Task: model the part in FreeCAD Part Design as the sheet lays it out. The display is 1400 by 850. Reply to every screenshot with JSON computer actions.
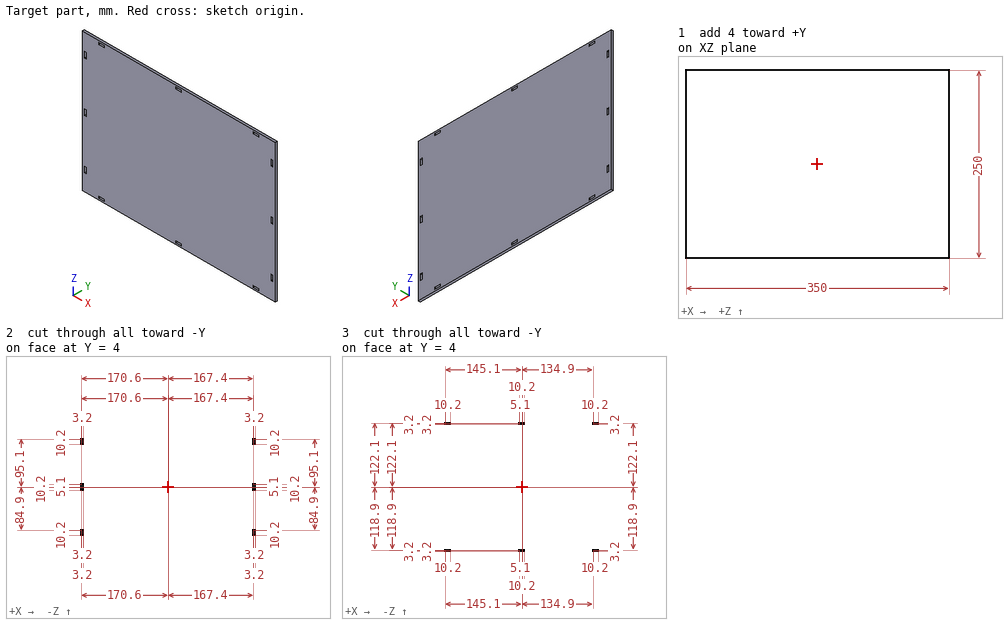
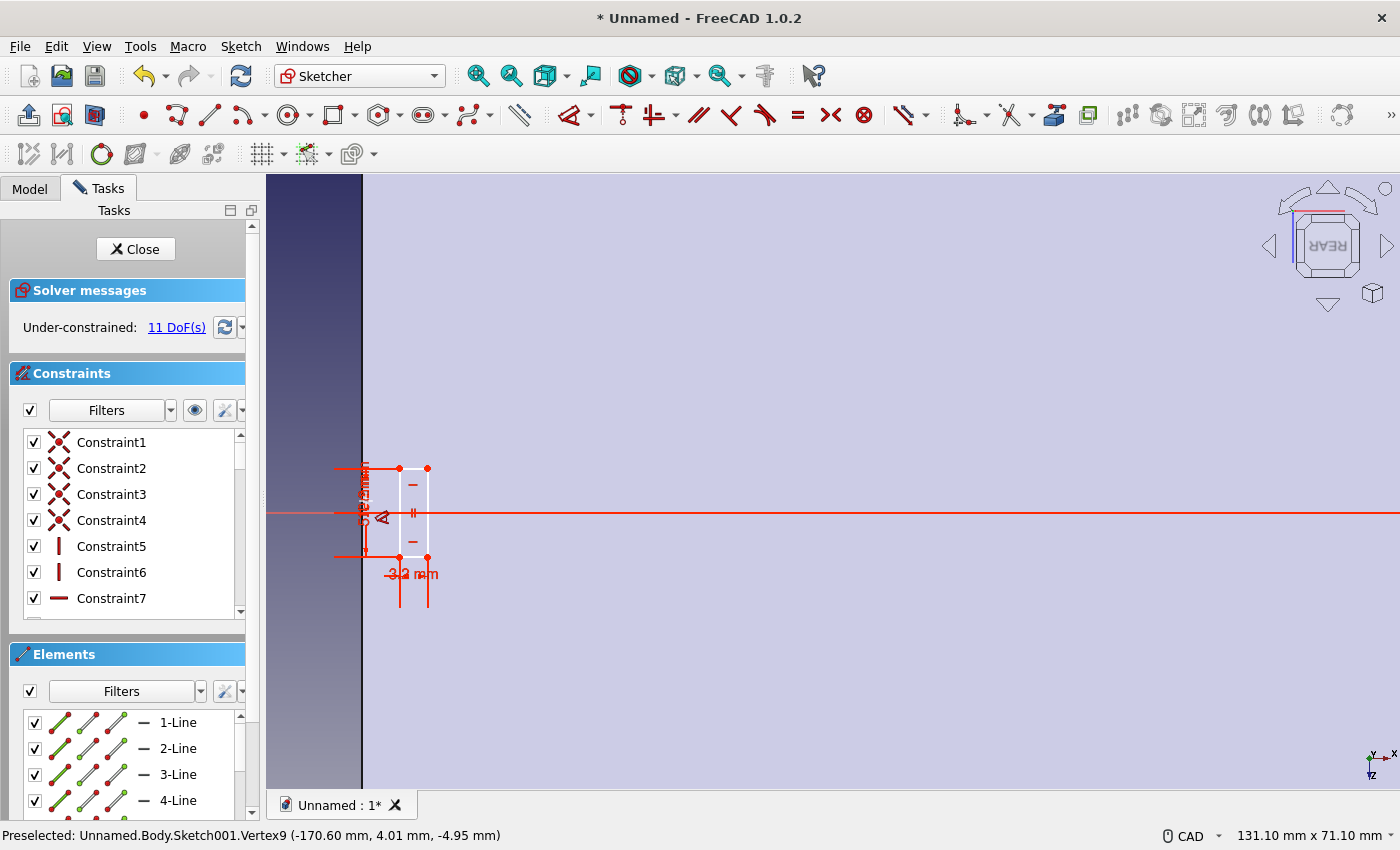
{"action": "scroll", "coordinate": [401, 471], "scroll_direction": "down", "scroll_amount": 7}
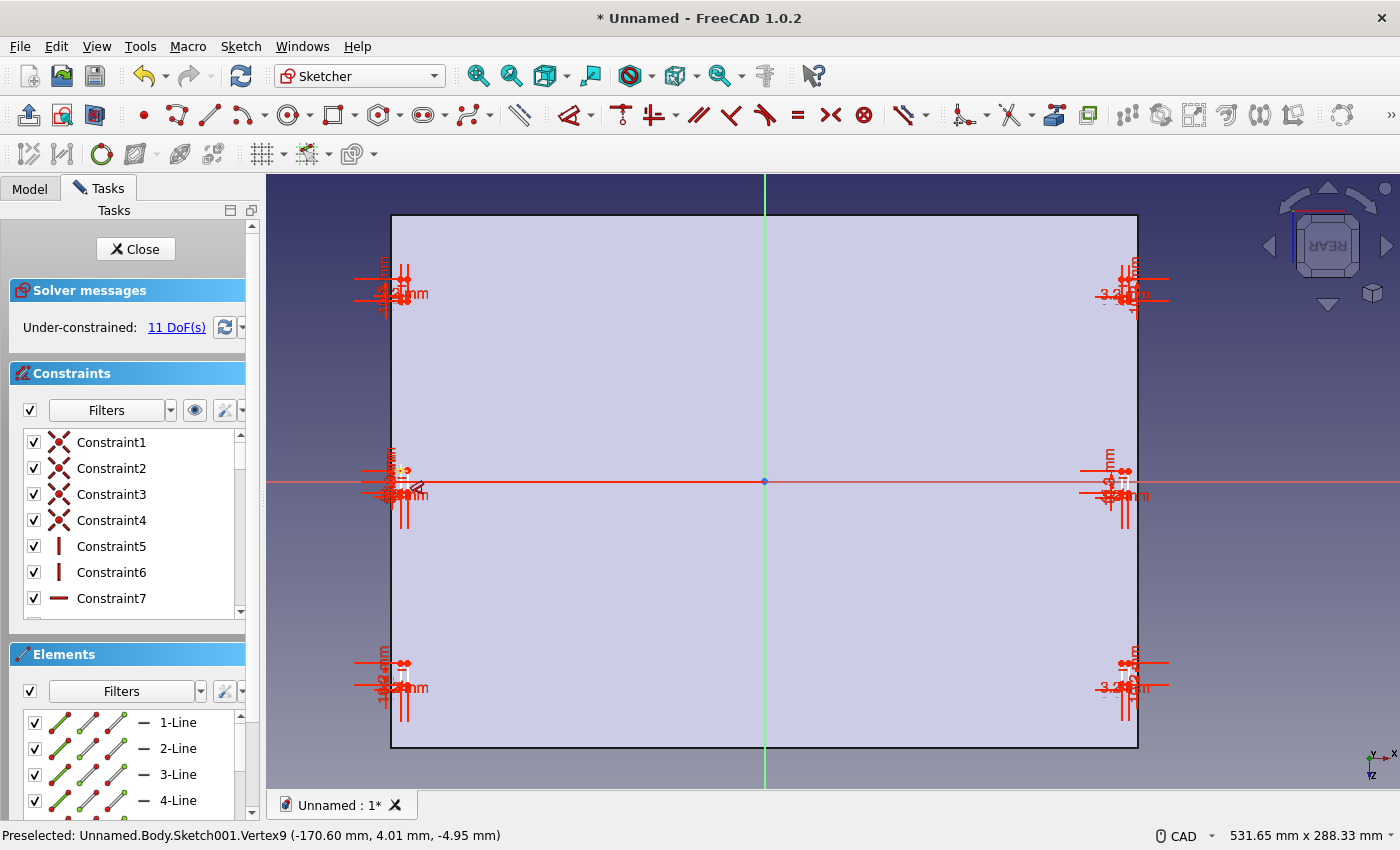
{"action": "scroll", "coordinate": [1122, 471], "scroll_direction": "up", "scroll_amount": 7}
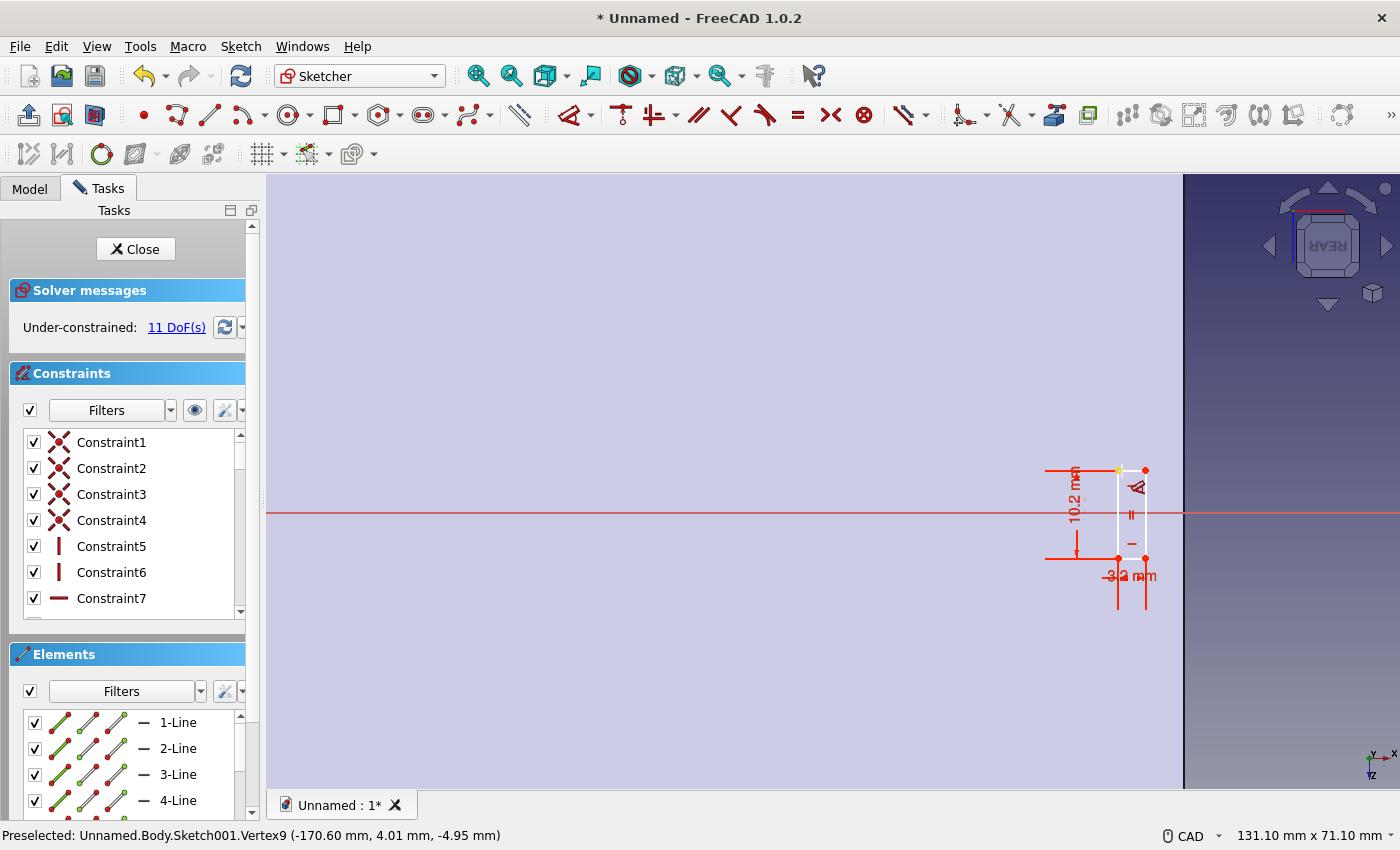
{"action": "left_click", "coordinate": [1118, 471]}
{"action": "left_click", "coordinate": [1176, 492]}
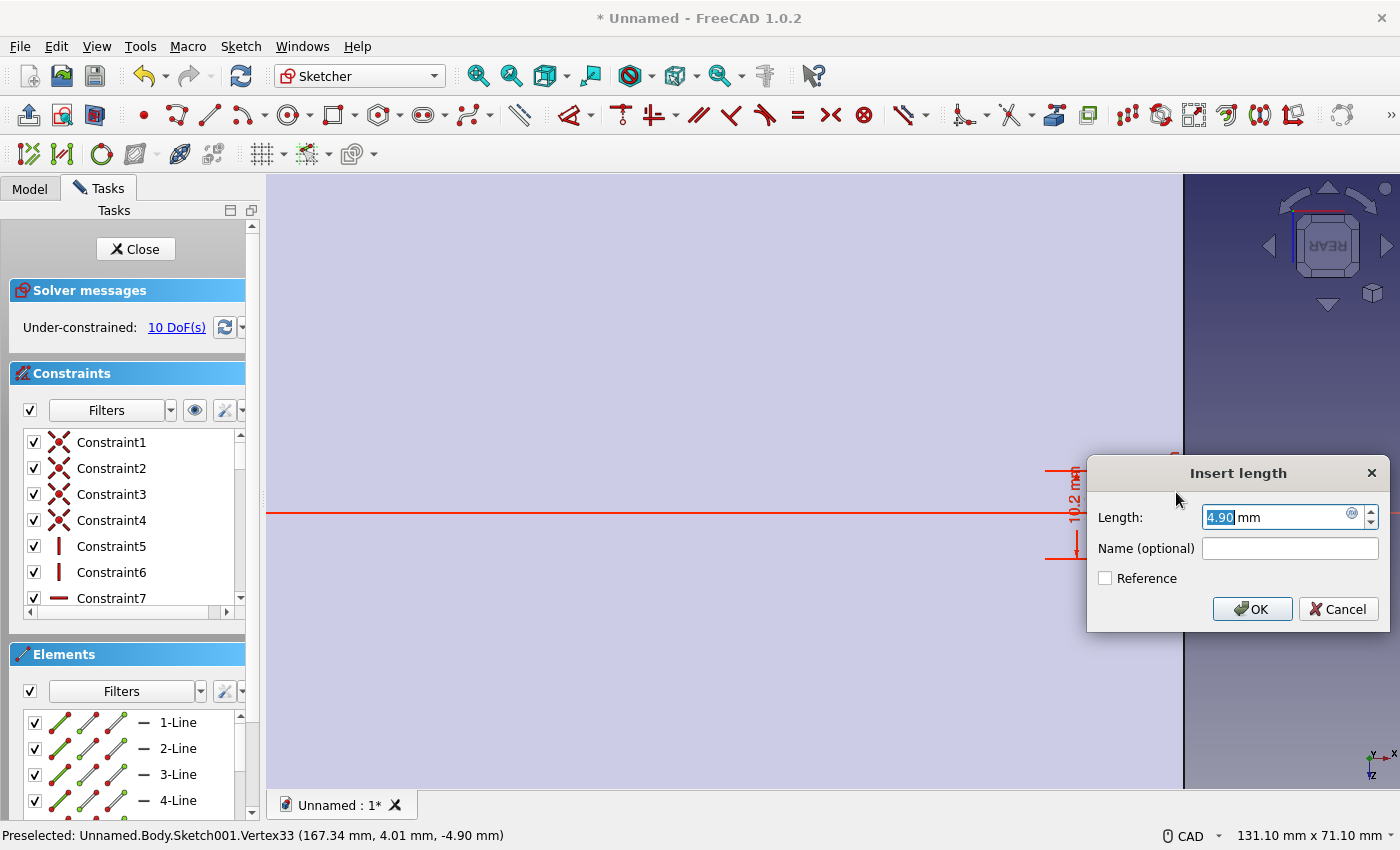
{"action": "type", "text": "5.1"}
{"action": "key", "text": "Return"}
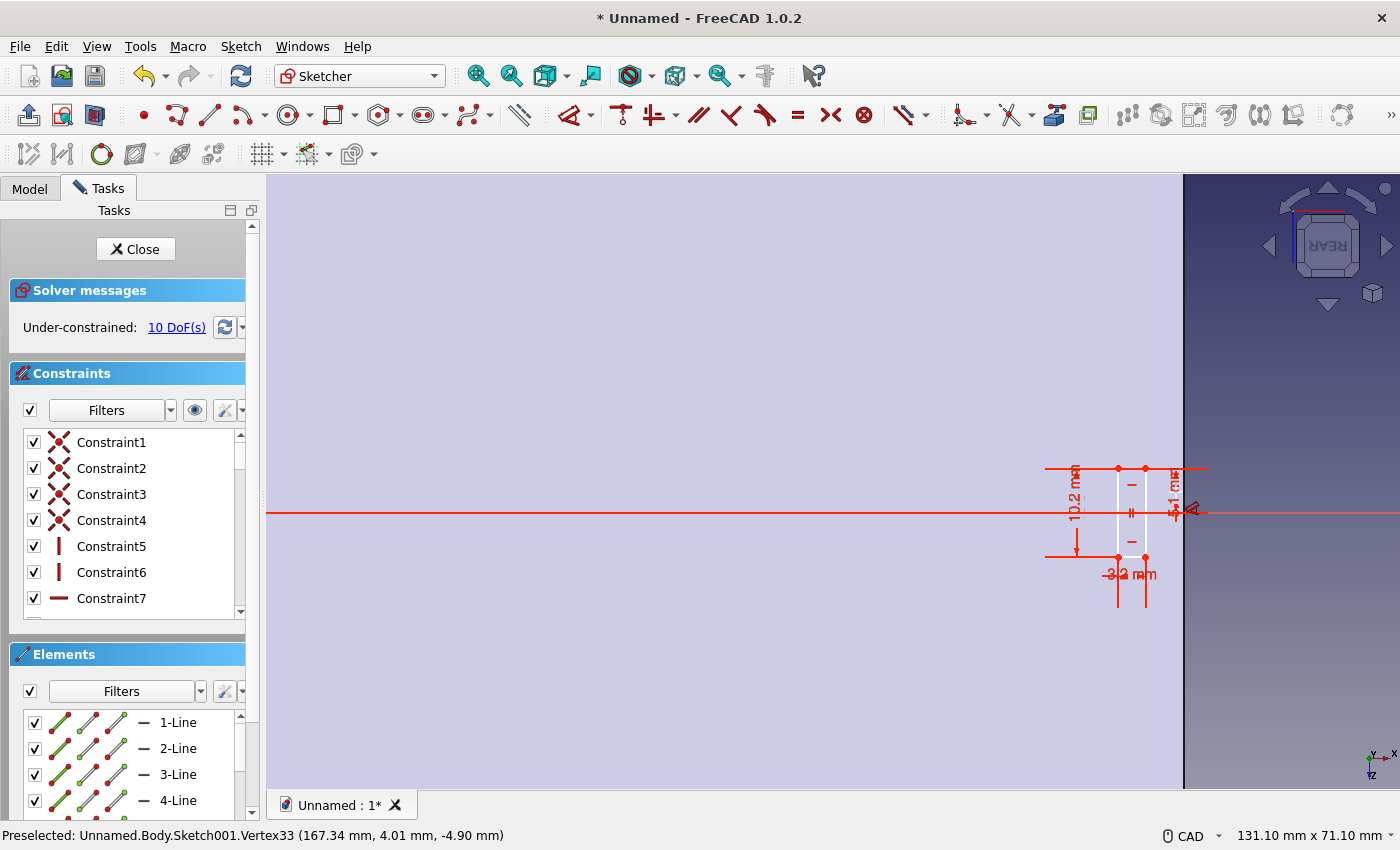
{"action": "scroll", "coordinate": [1122, 471], "scroll_direction": "down", "scroll_amount": 7}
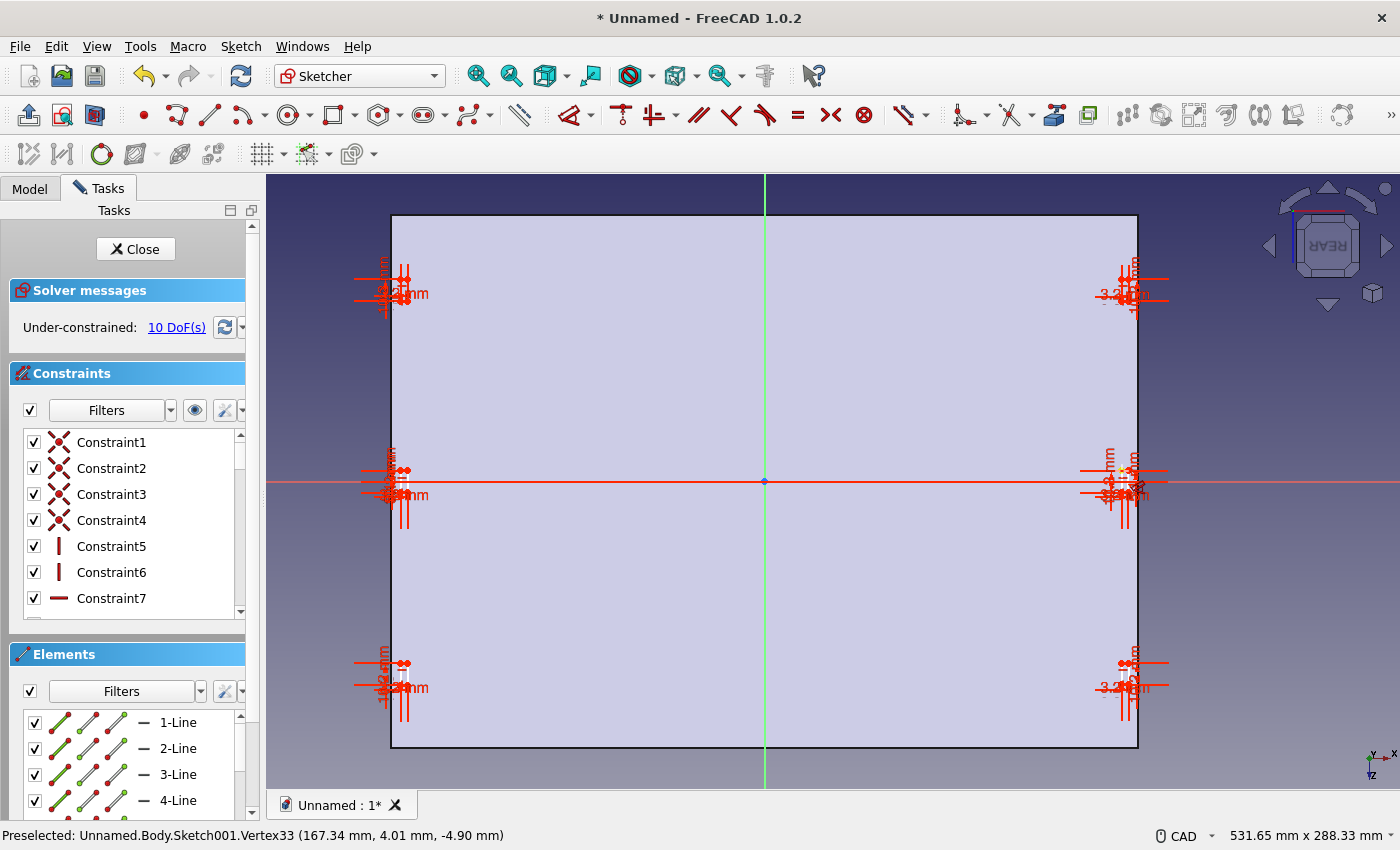
{"action": "scroll", "coordinate": [401, 279], "scroll_direction": "up", "scroll_amount": 3}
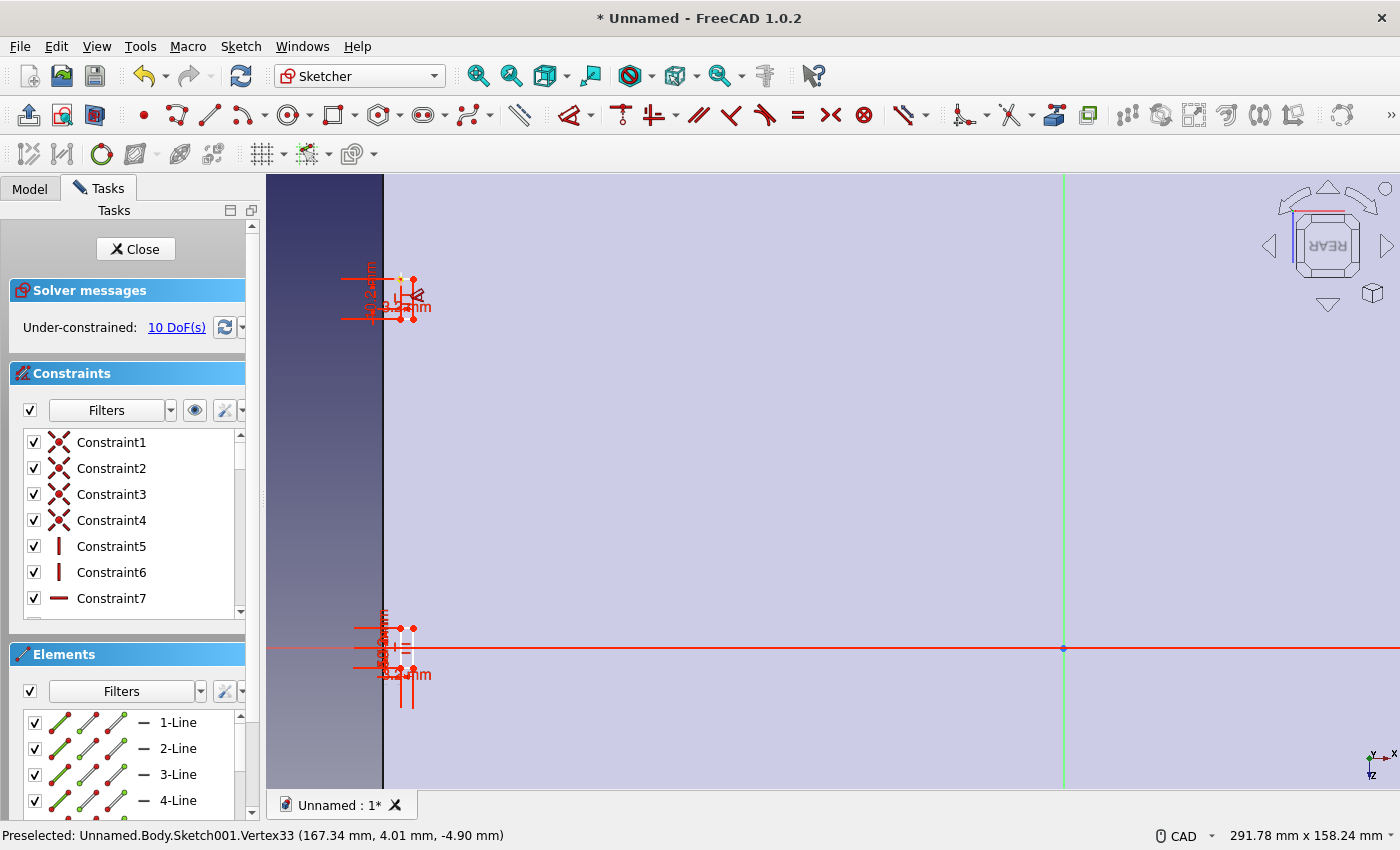
{"action": "left_click", "coordinate": [401, 279]}
{"action": "left_click", "coordinate": [367, 464]}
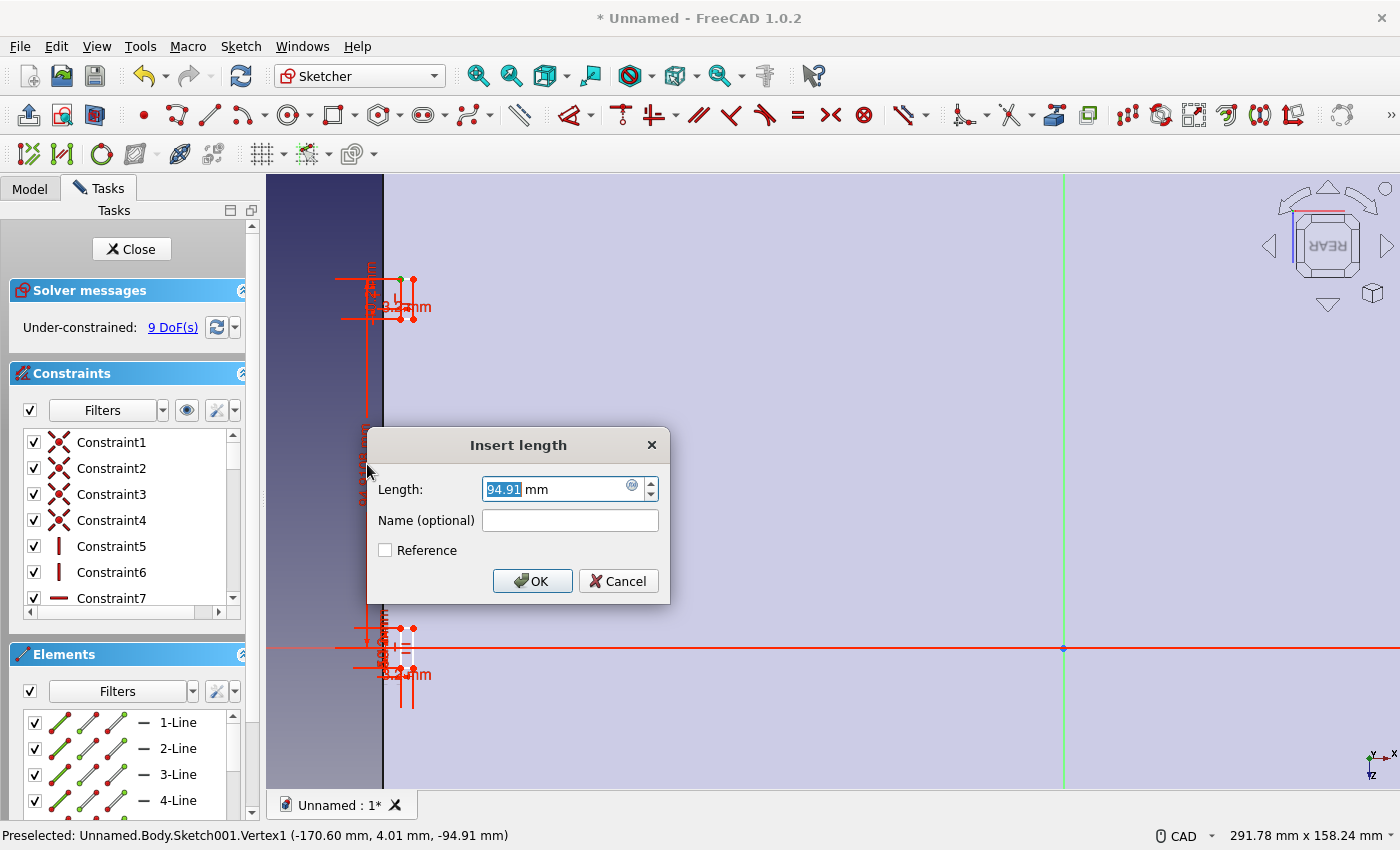
{"action": "type", "text": "95.1"}
{"action": "key", "text": "Return"}